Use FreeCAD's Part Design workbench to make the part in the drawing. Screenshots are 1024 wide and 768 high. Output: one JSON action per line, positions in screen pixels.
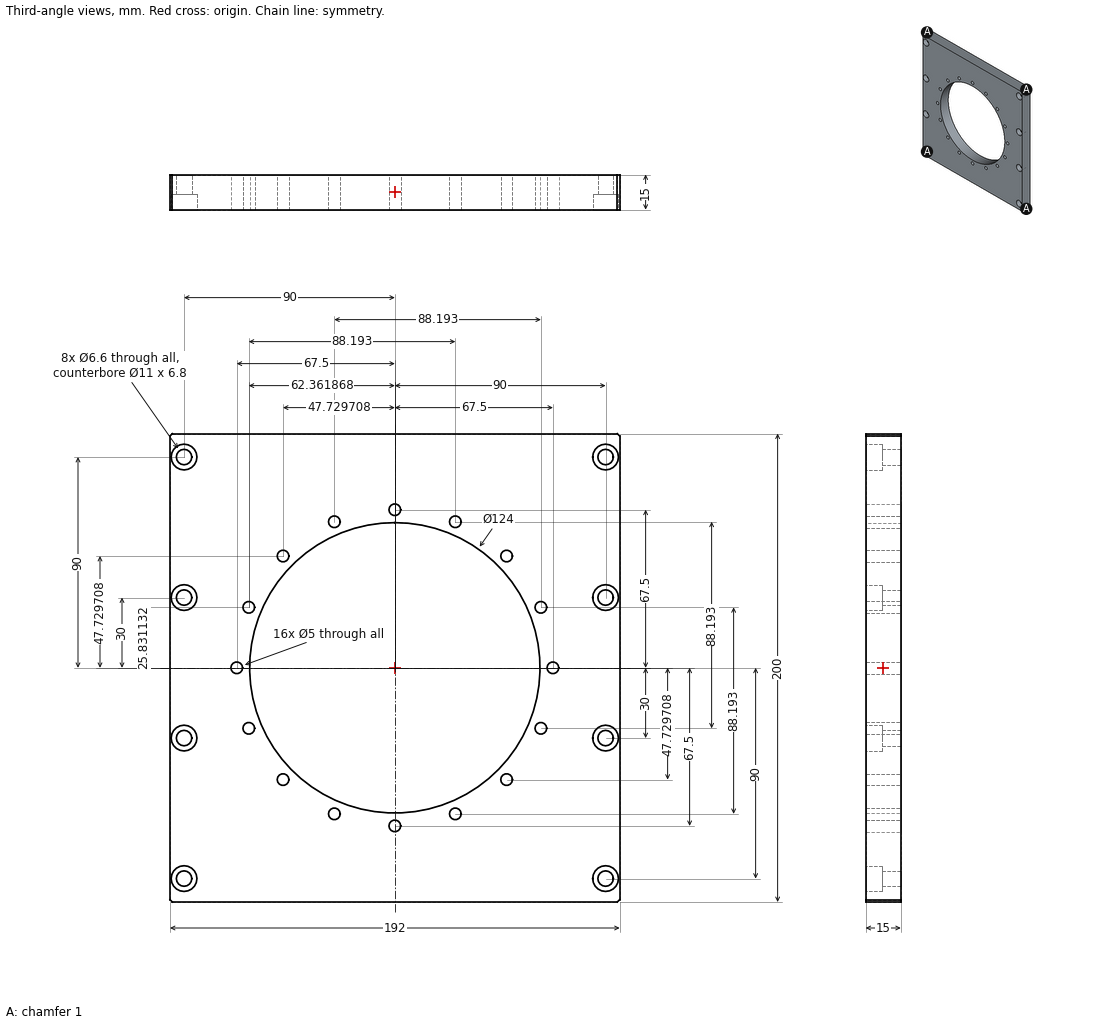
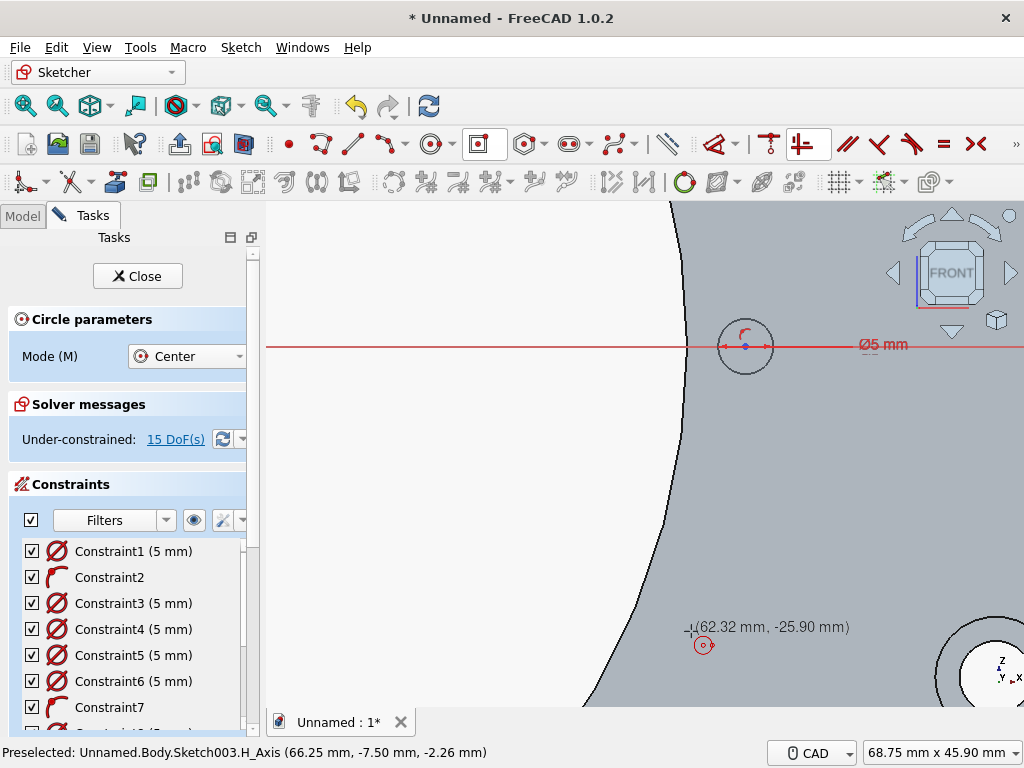
{"action": "scroll", "coordinate": [721, 481], "scroll_direction": "down", "scroll_amount": 8}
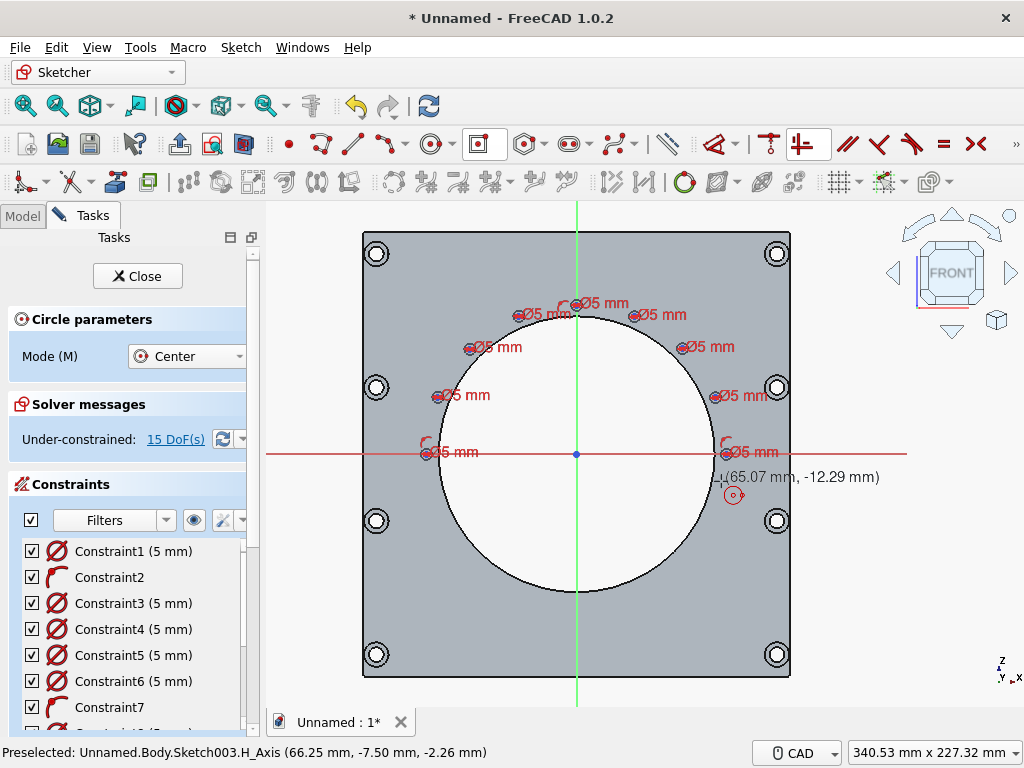
{"action": "left_click", "coordinate": [715, 512]}
{"action": "mouse_move", "coordinate": [719, 508]}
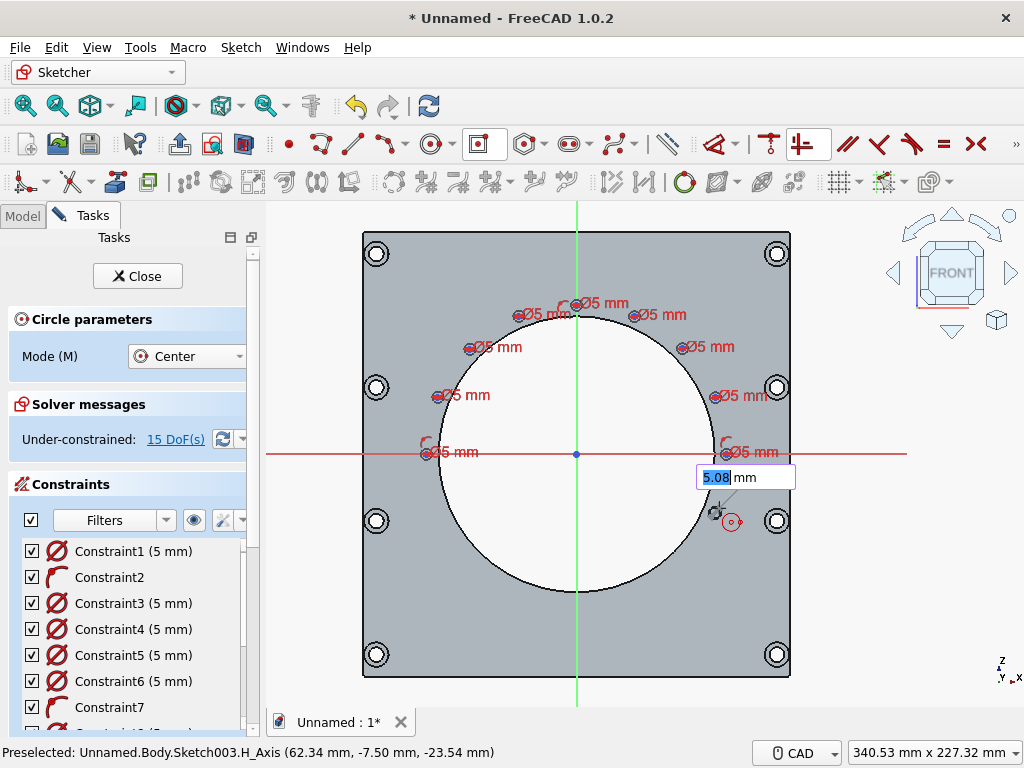
{"action": "type", "text": "5"}
{"action": "key", "text": "Return"}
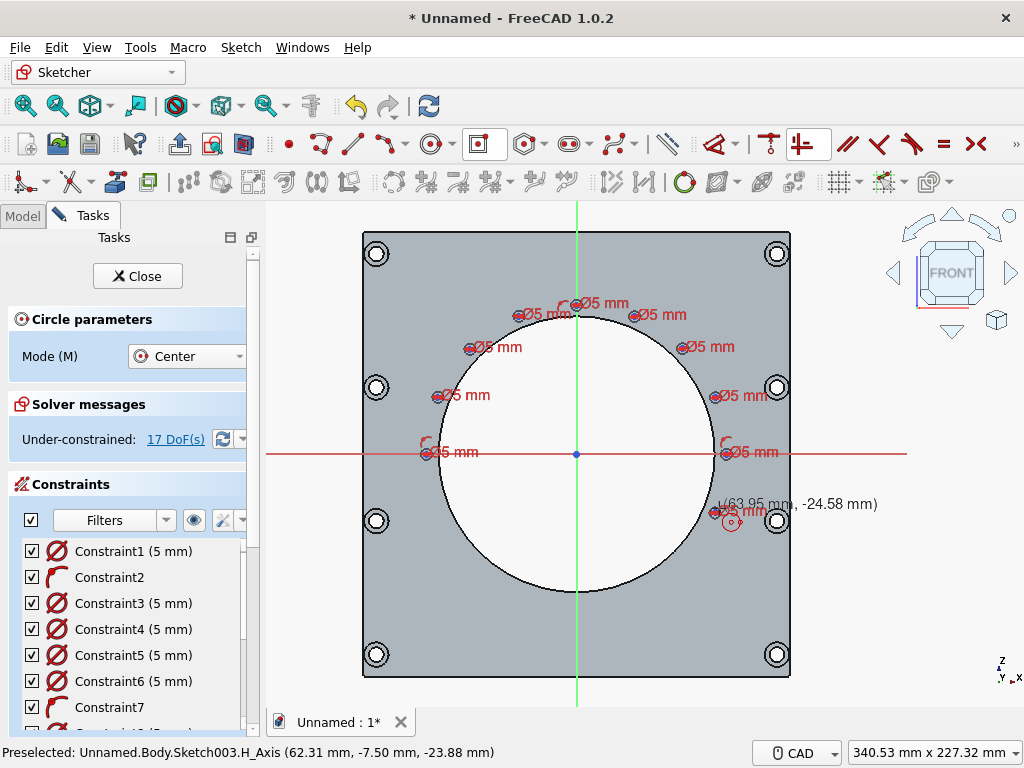
{"action": "scroll", "coordinate": [683, 561], "scroll_direction": "up", "scroll_amount": 8}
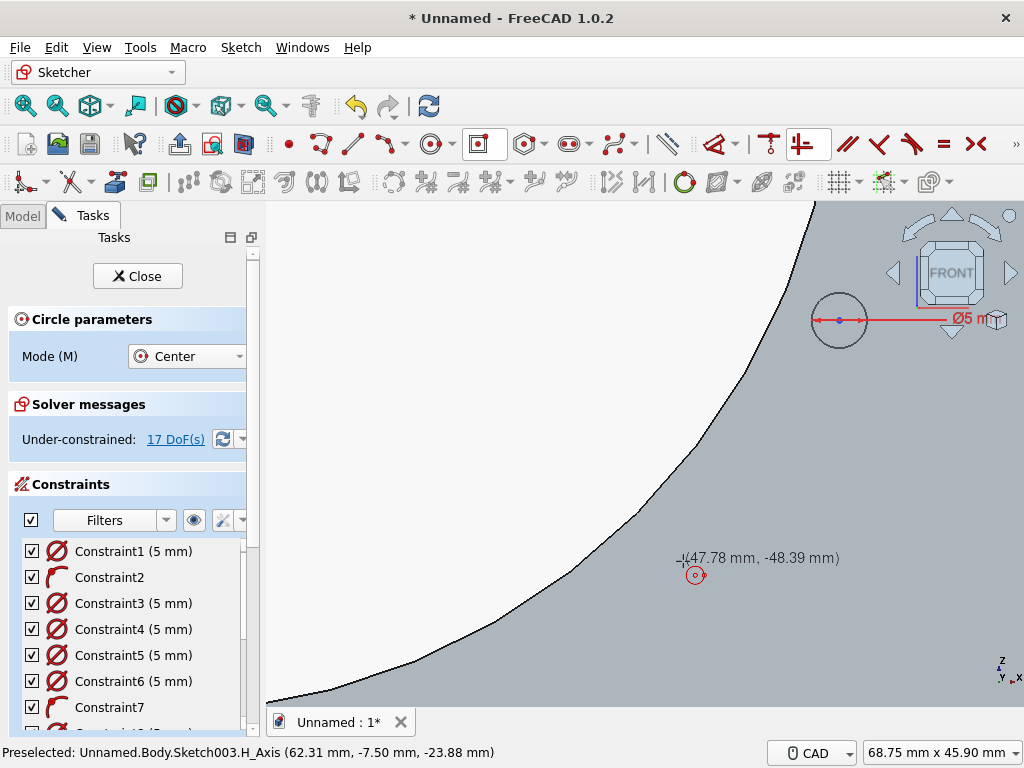
{"action": "scroll", "coordinate": [683, 561], "scroll_direction": "down", "scroll_amount": 8}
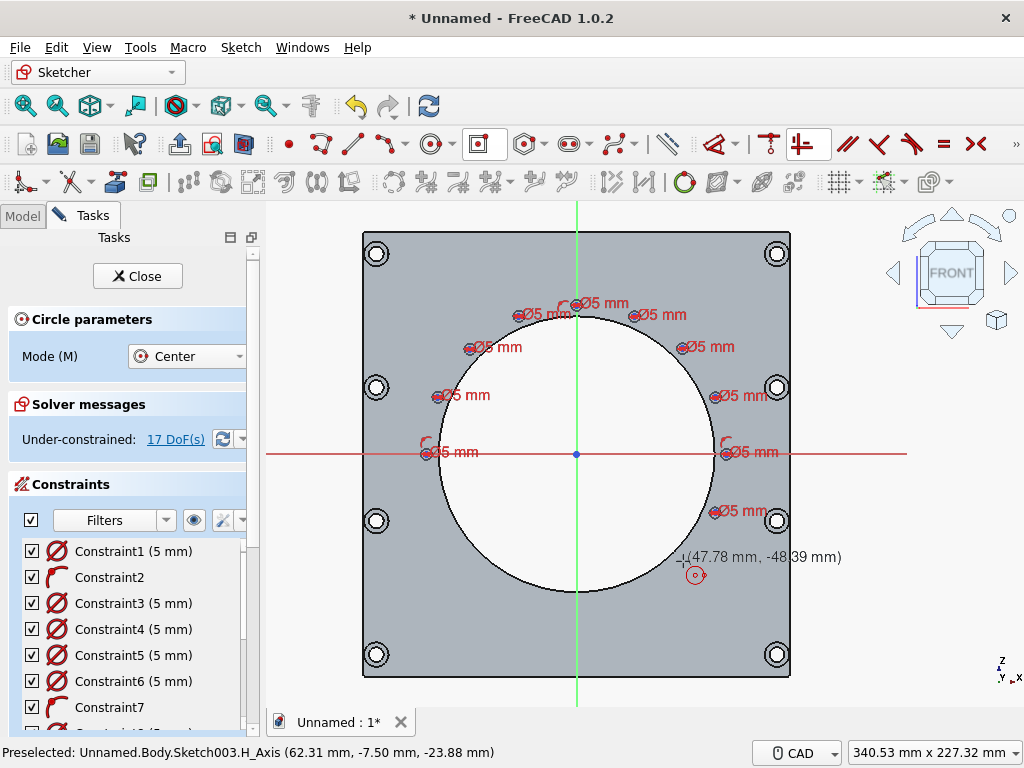
{"action": "left_click", "coordinate": [683, 561]}
{"action": "mouse_move", "coordinate": [687, 557]}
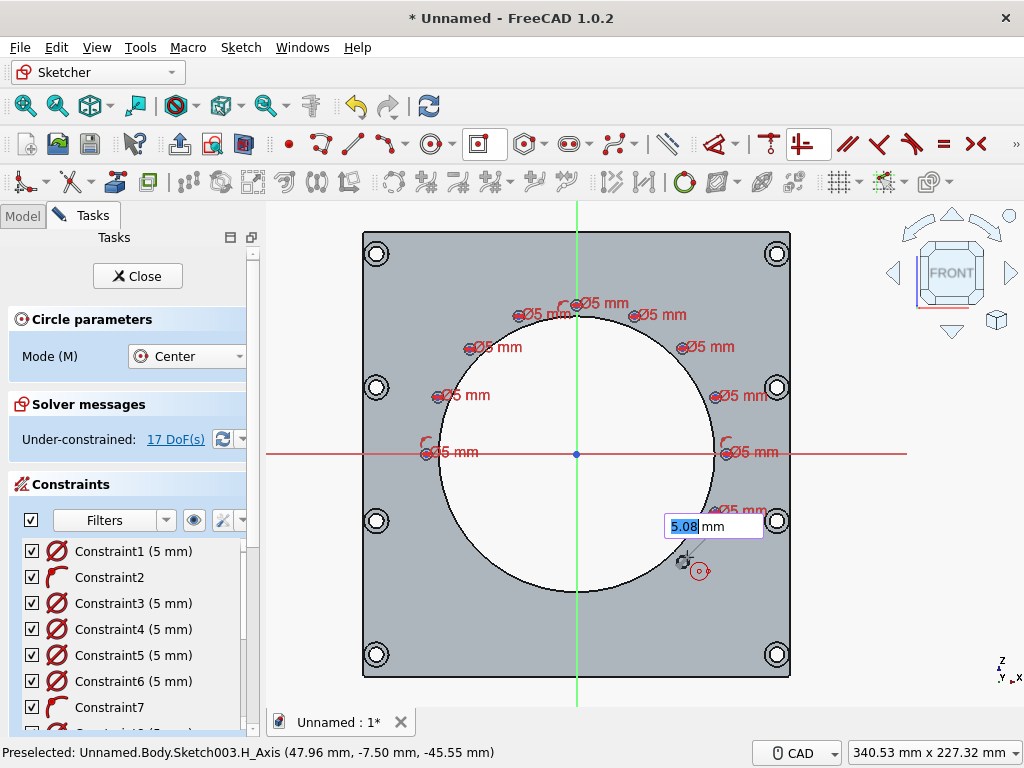
{"action": "type", "text": "5"}
{"action": "key", "text": "Return"}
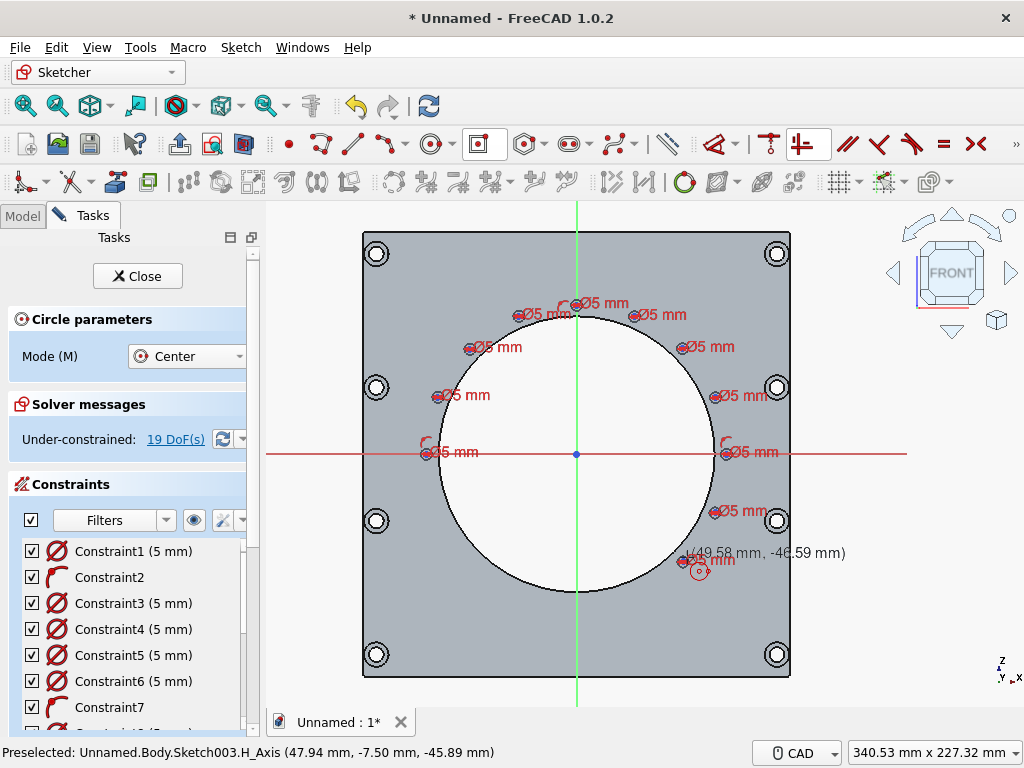
{"action": "scroll", "coordinate": [634, 593], "scroll_direction": "up", "scroll_amount": 8}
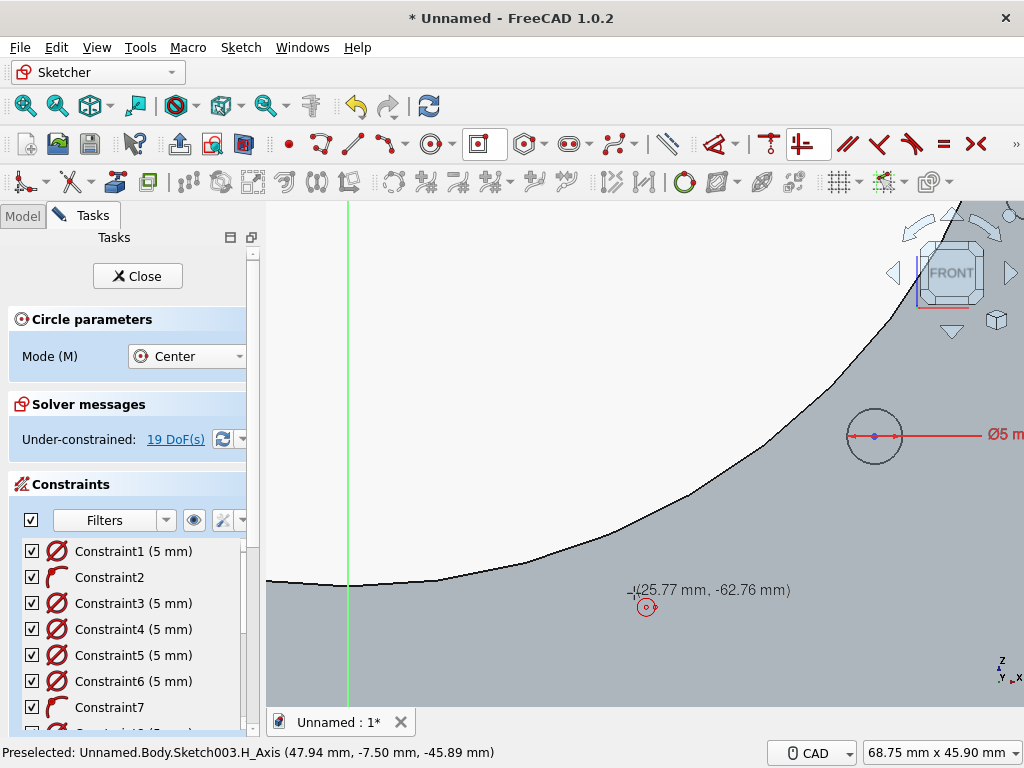
{"action": "scroll", "coordinate": [634, 593], "scroll_direction": "down", "scroll_amount": 8}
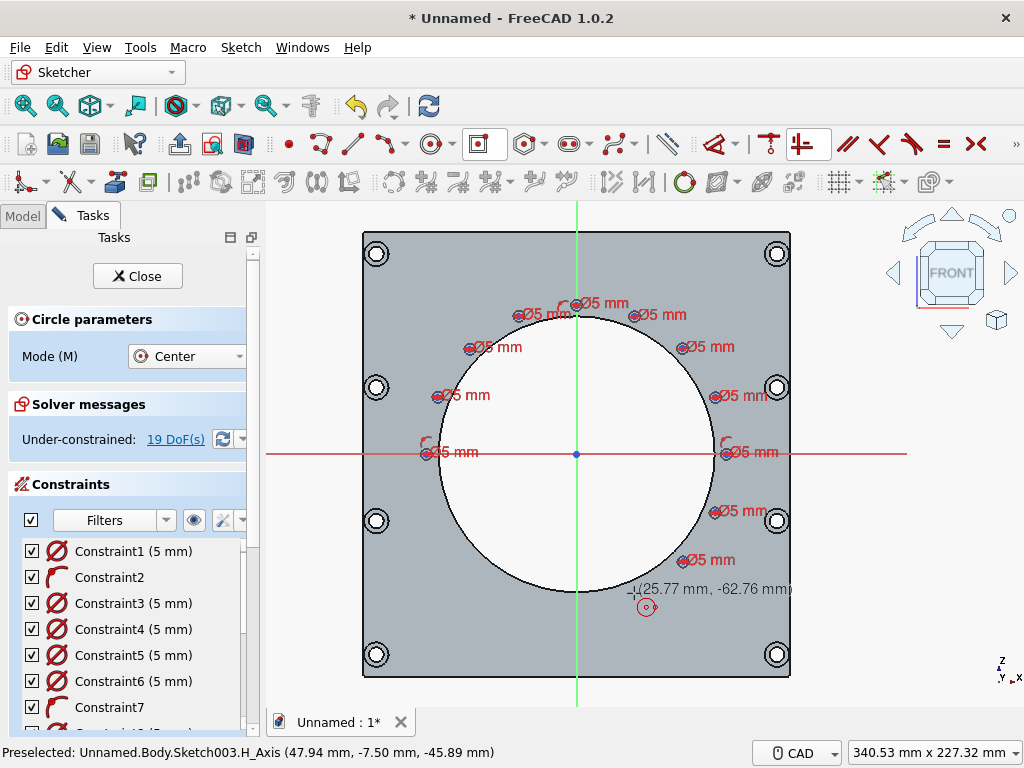
{"action": "left_click", "coordinate": [634, 593]}
{"action": "mouse_move", "coordinate": [638, 589]}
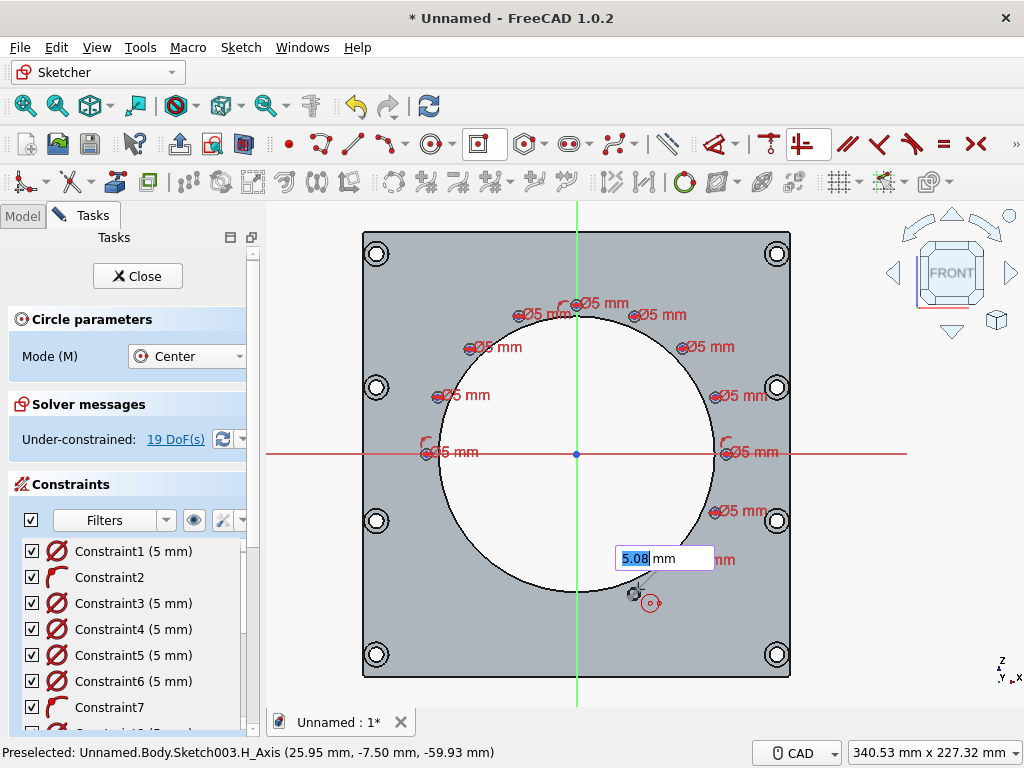
{"action": "type", "text": "5"}
{"action": "key", "text": "Return"}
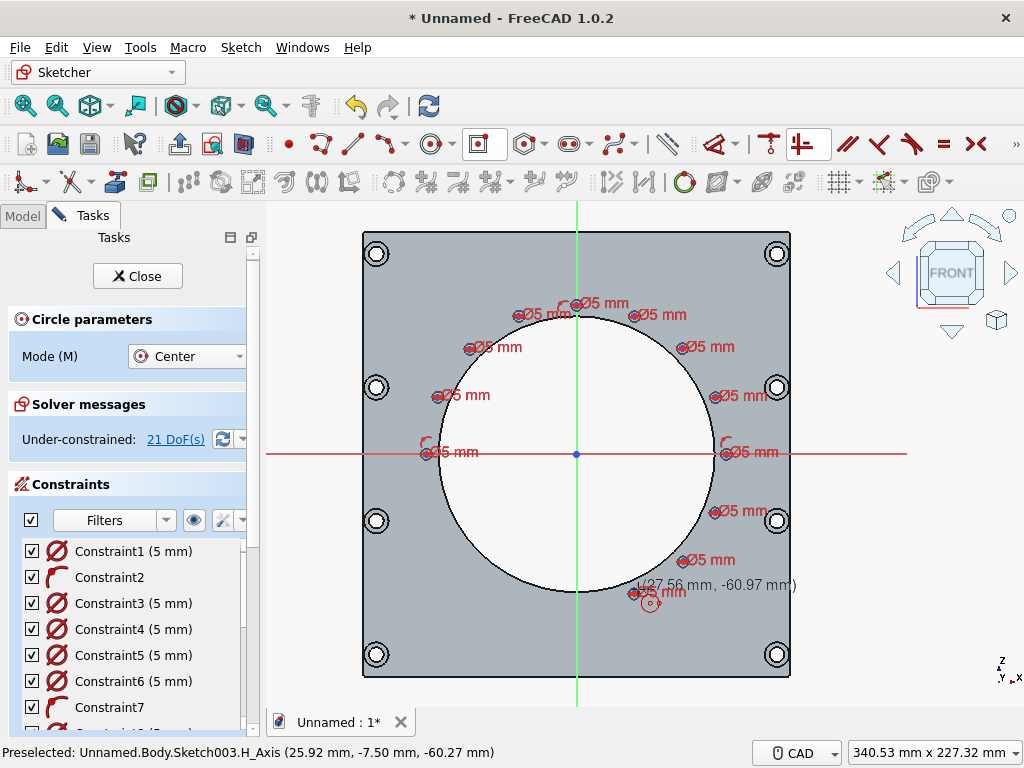
{"action": "scroll", "coordinate": [577, 605], "scroll_direction": "up", "scroll_amount": 8}